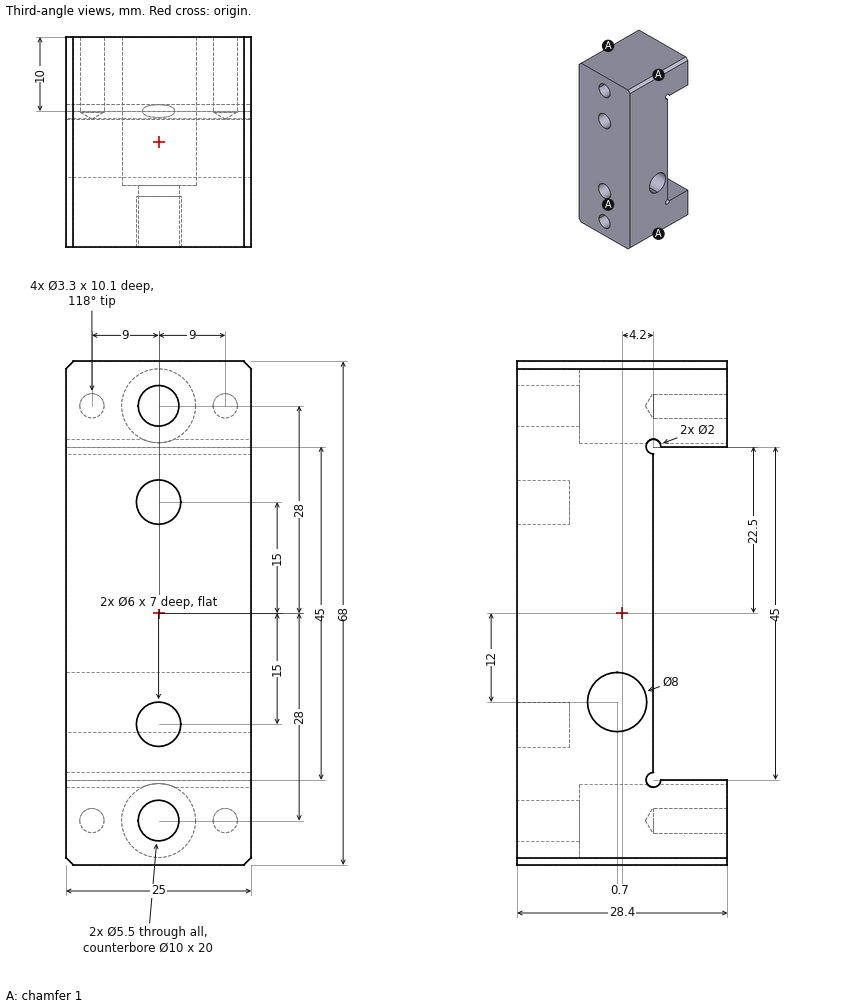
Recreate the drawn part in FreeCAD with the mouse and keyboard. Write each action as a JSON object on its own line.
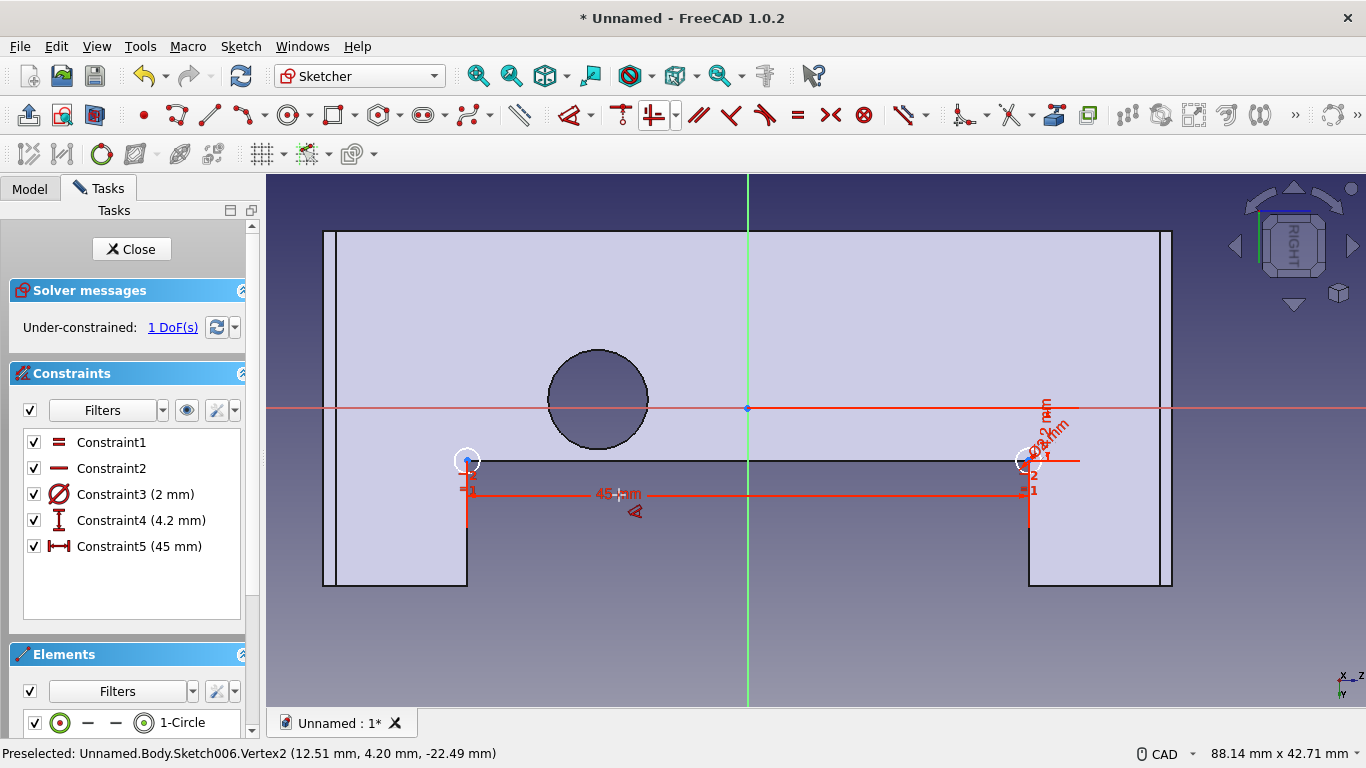
{"action": "left_click", "coordinate": [1029, 461]}
{"action": "left_click", "coordinate": [888, 374]}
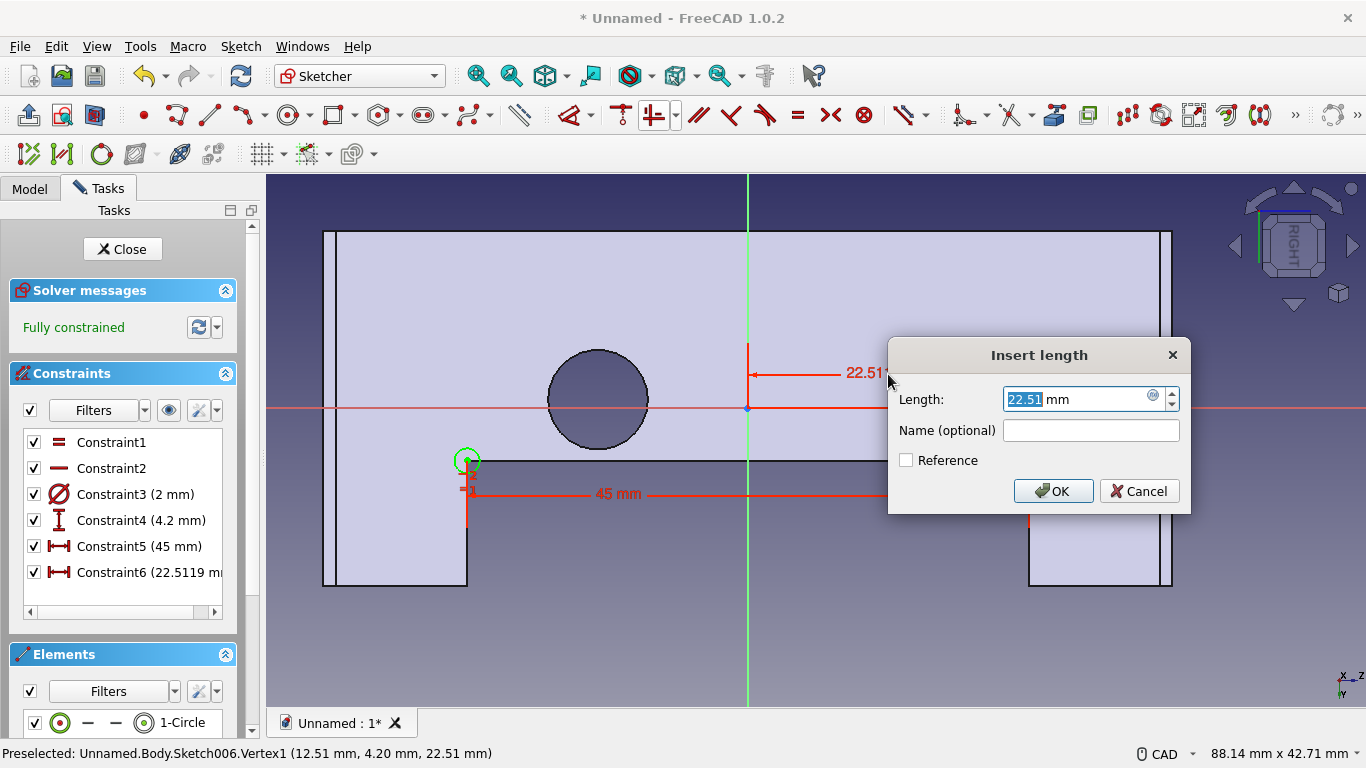
{"action": "type", "text": "22.5"}
{"action": "key", "text": "Return"}
{"action": "key", "text": "Escape"}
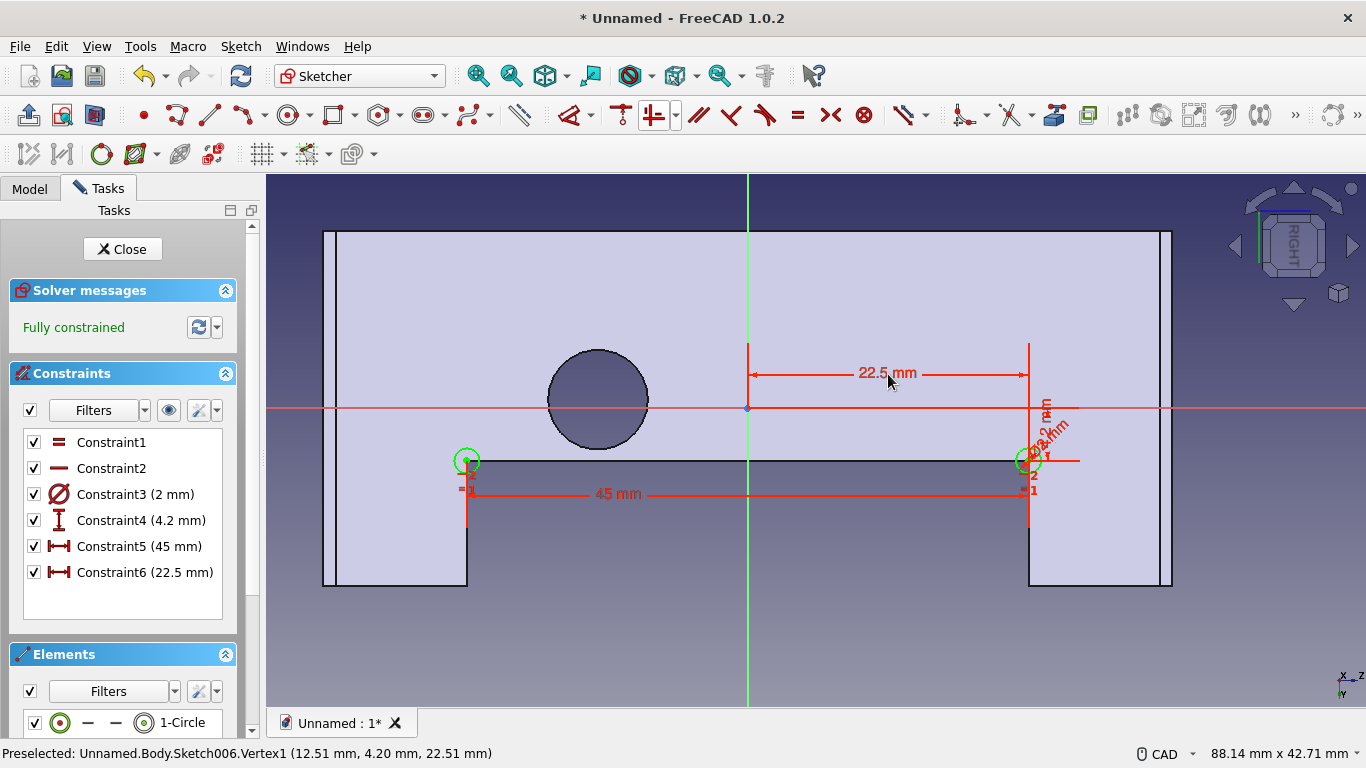
{"action": "left_click", "coordinate": [123, 249]}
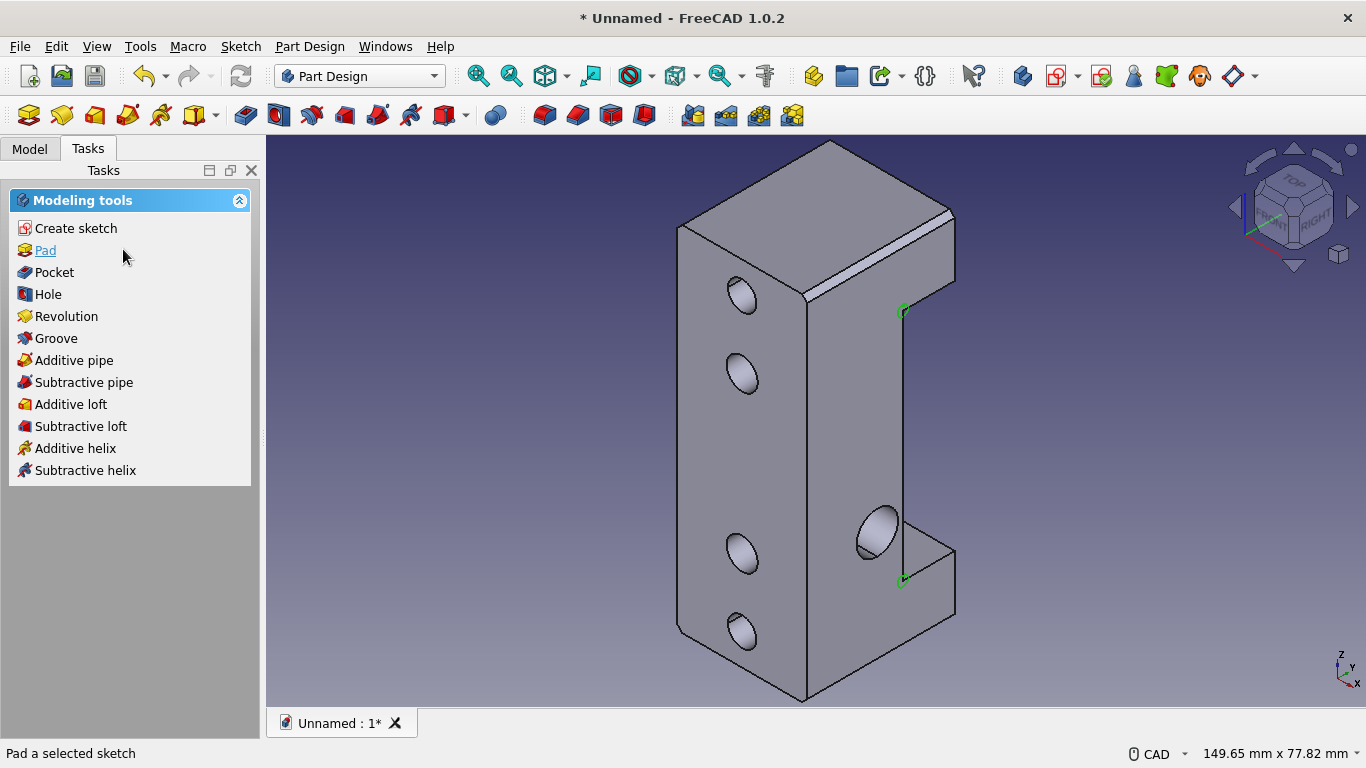
{"action": "left_click", "coordinate": [246, 116]}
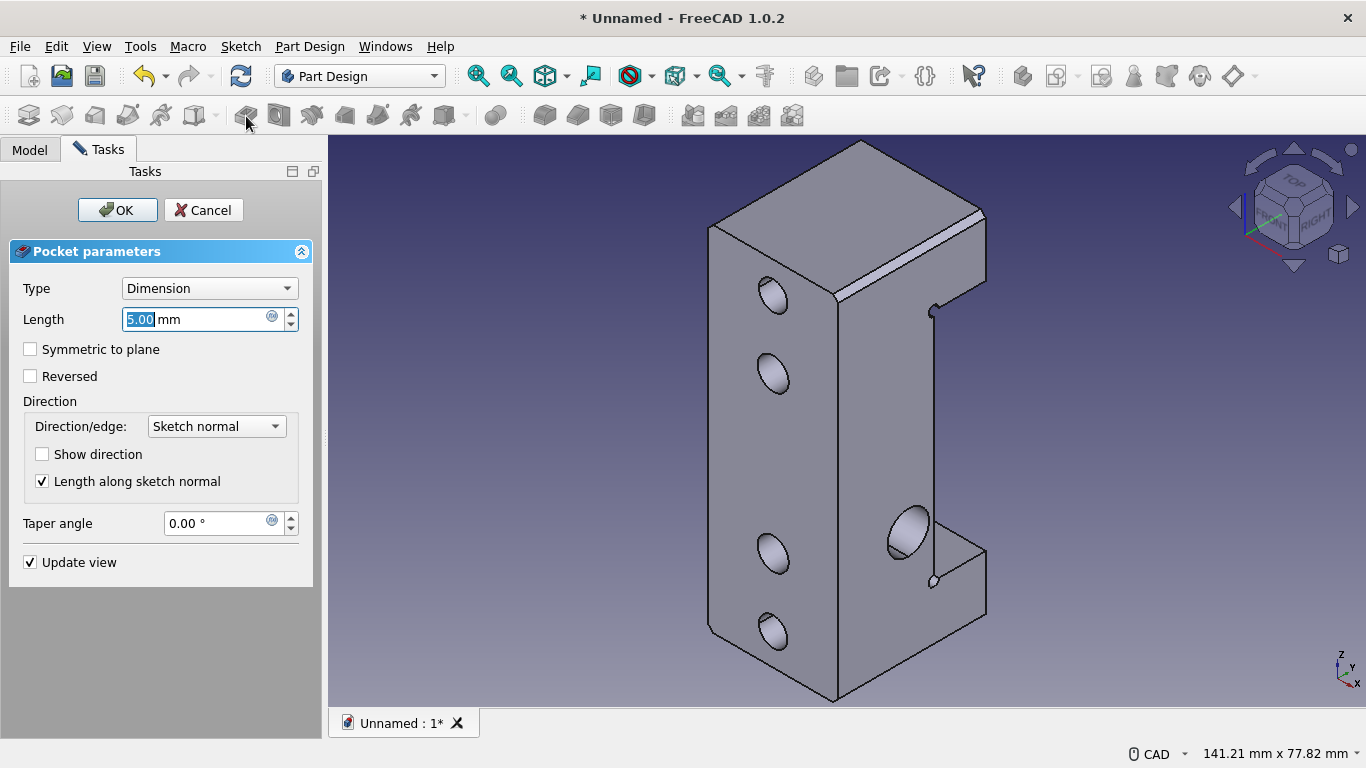
{"action": "left_click", "coordinate": [210, 288]}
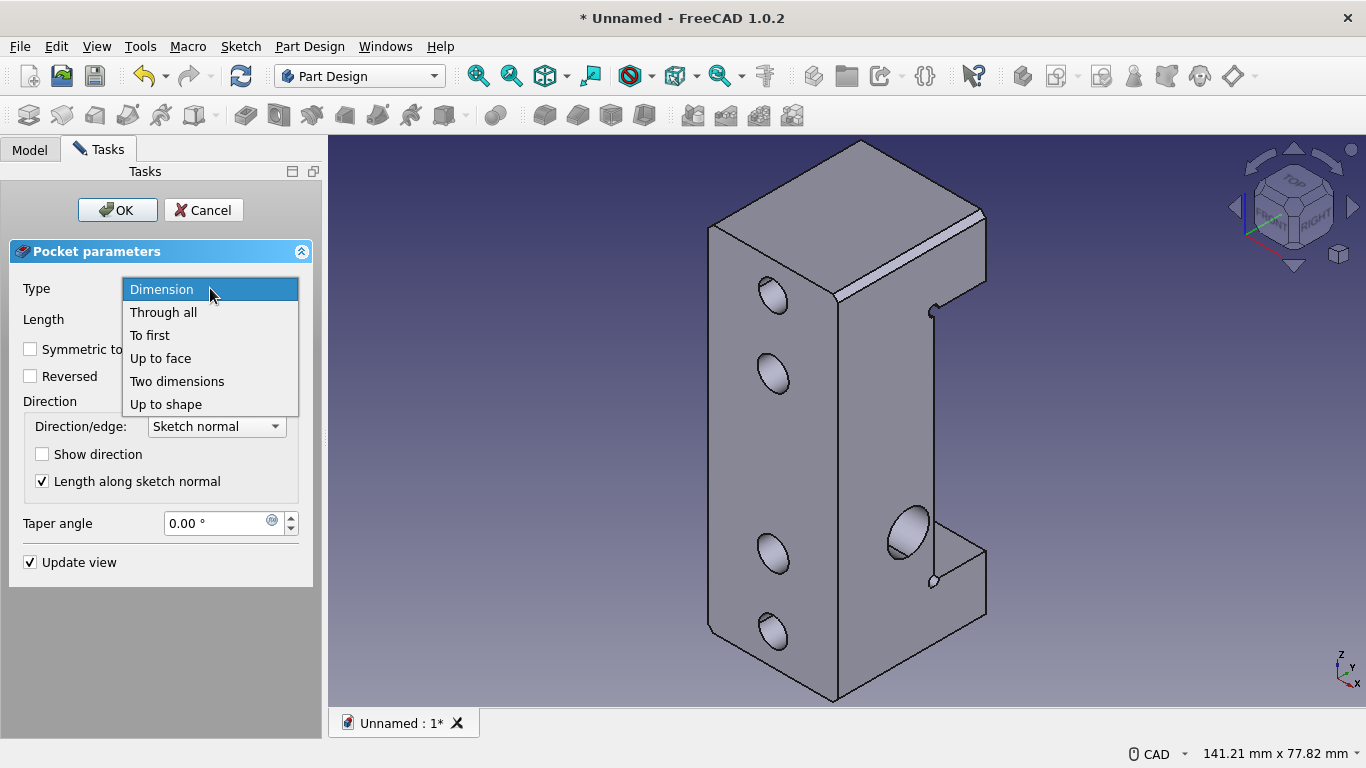
{"action": "left_click", "coordinate": [208, 312]}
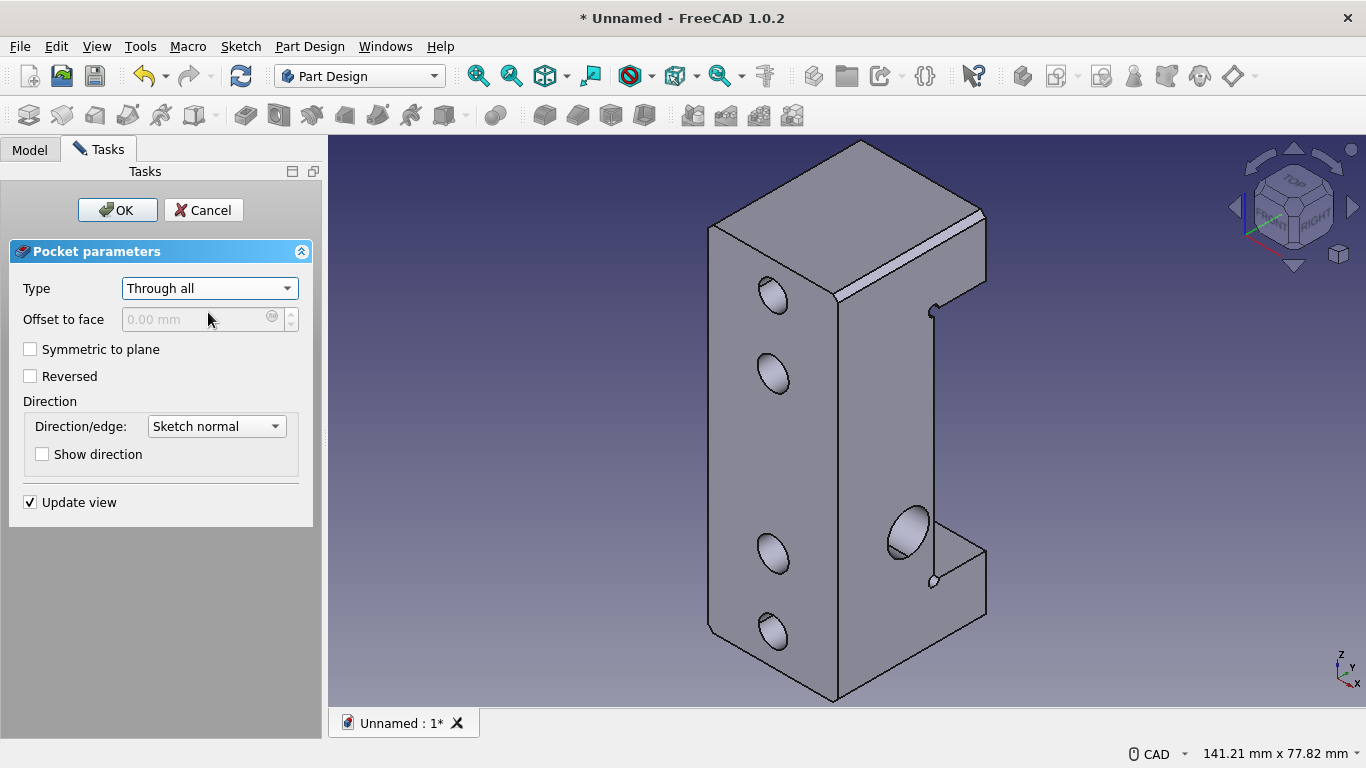
{"action": "left_click", "coordinate": [118, 210]}